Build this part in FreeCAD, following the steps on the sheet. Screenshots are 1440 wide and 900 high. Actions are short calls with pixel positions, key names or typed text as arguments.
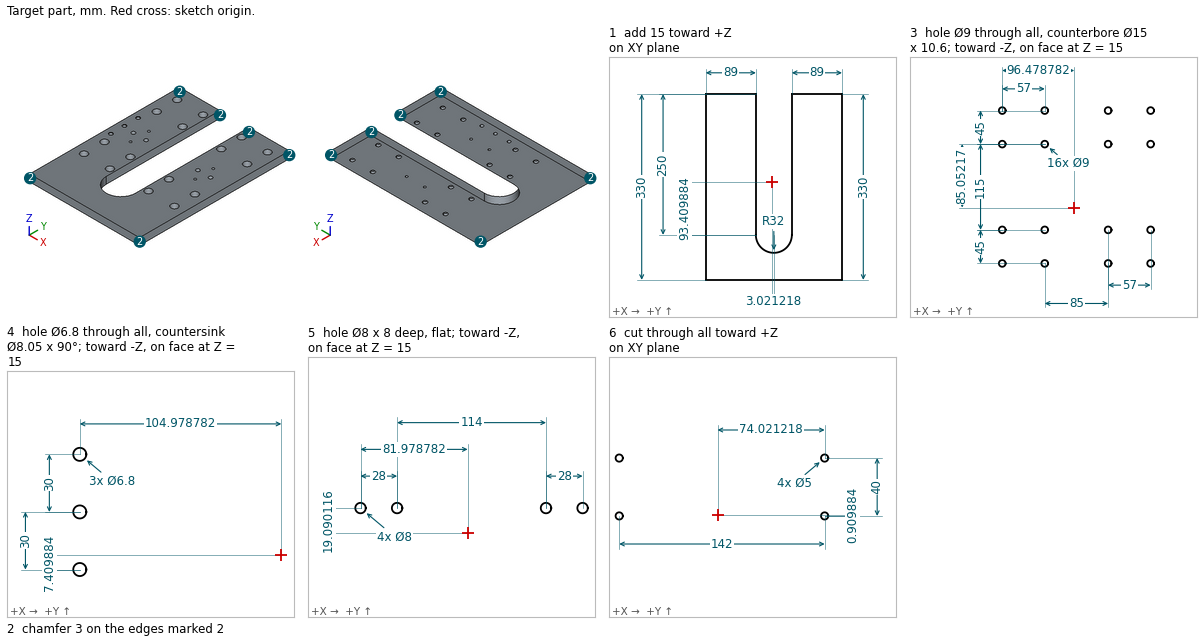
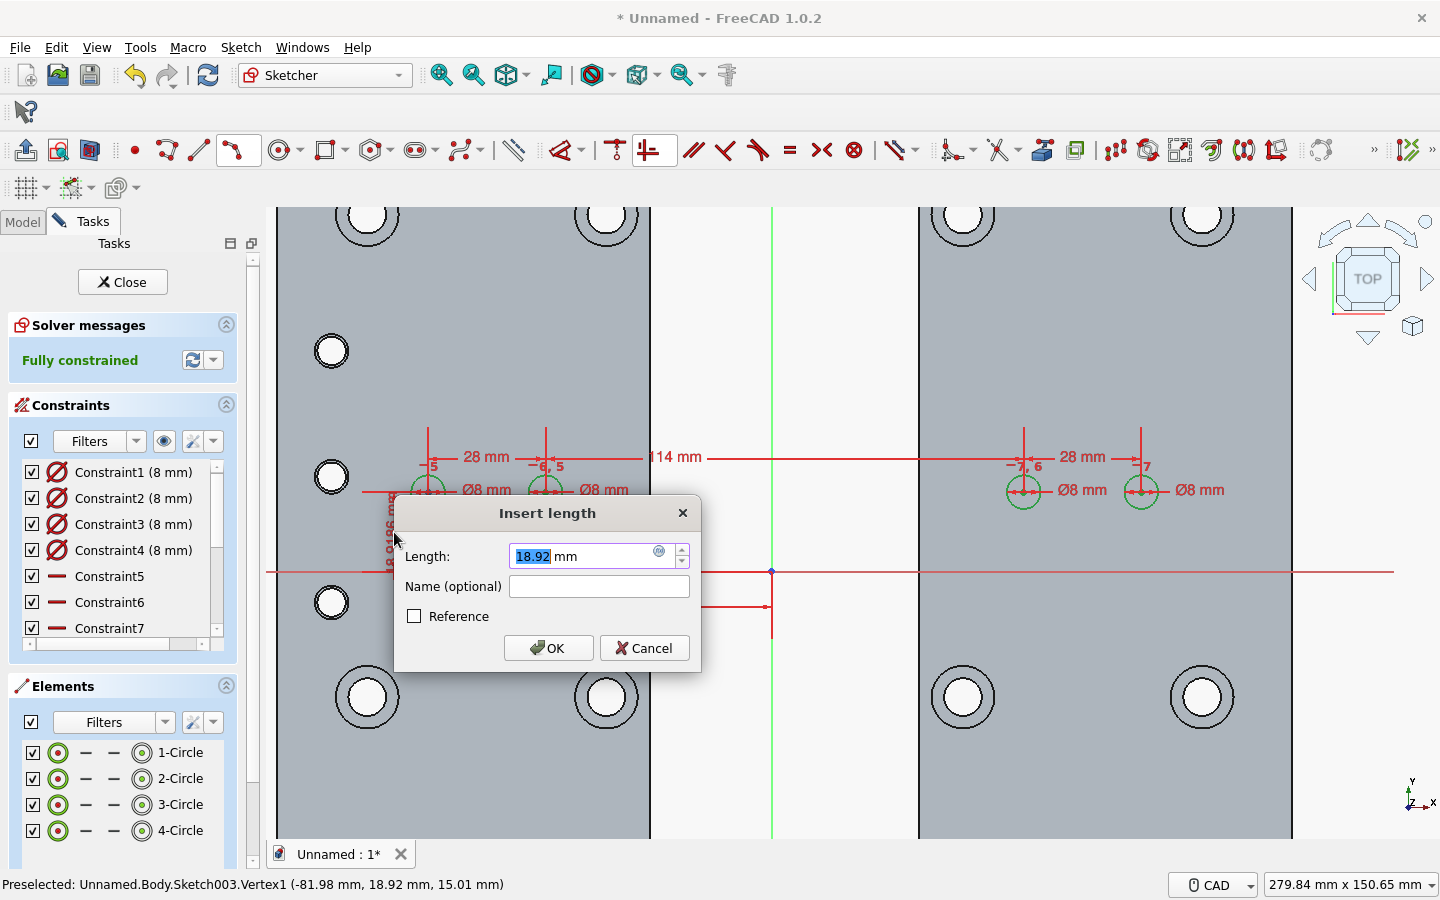
text(19.090116)
key(Return)
key(Escape)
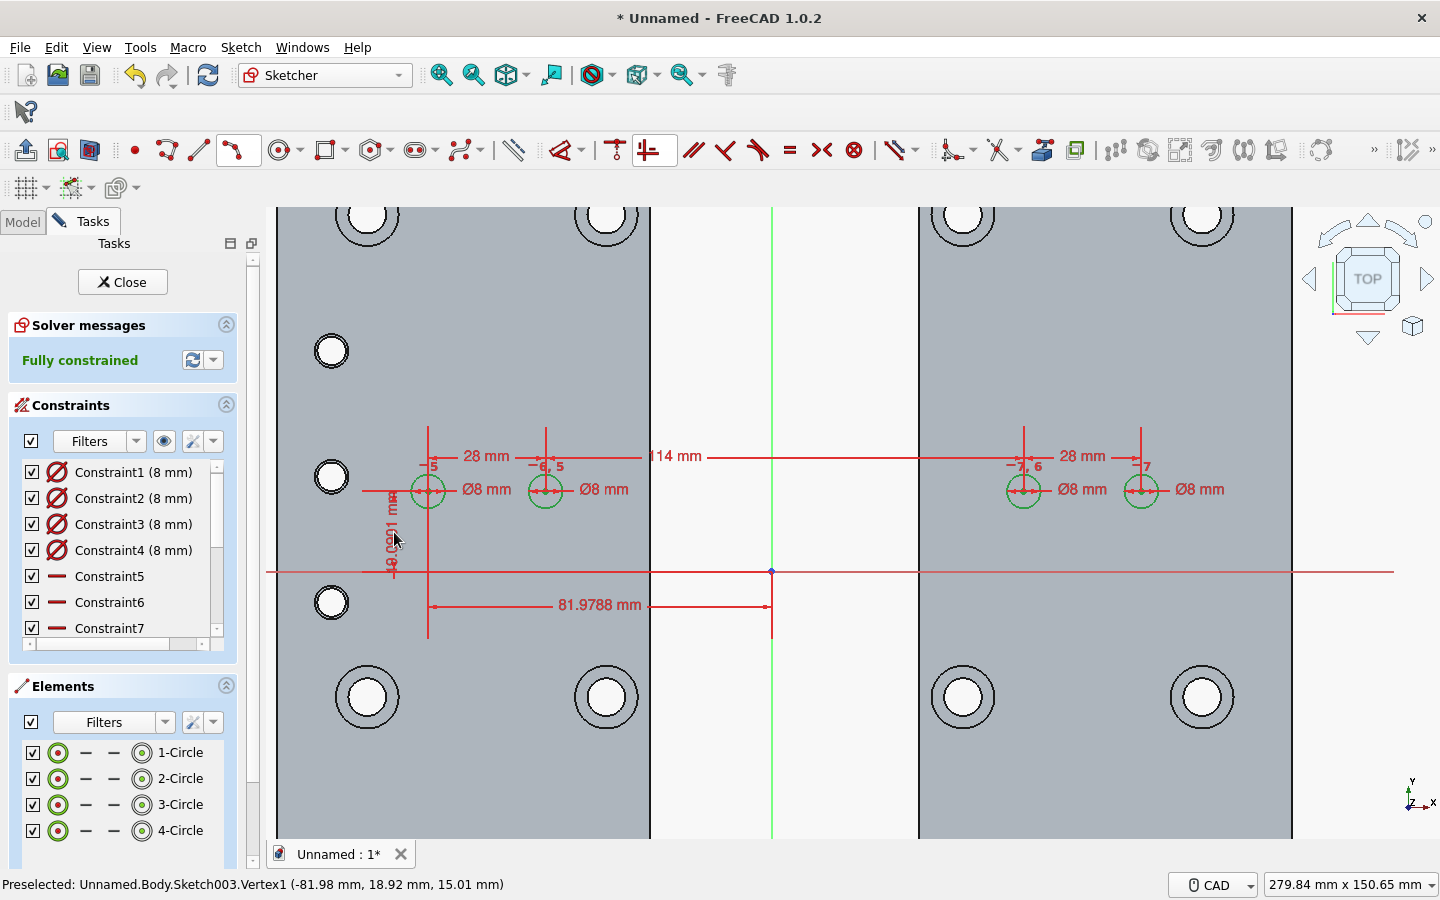
click(123, 282)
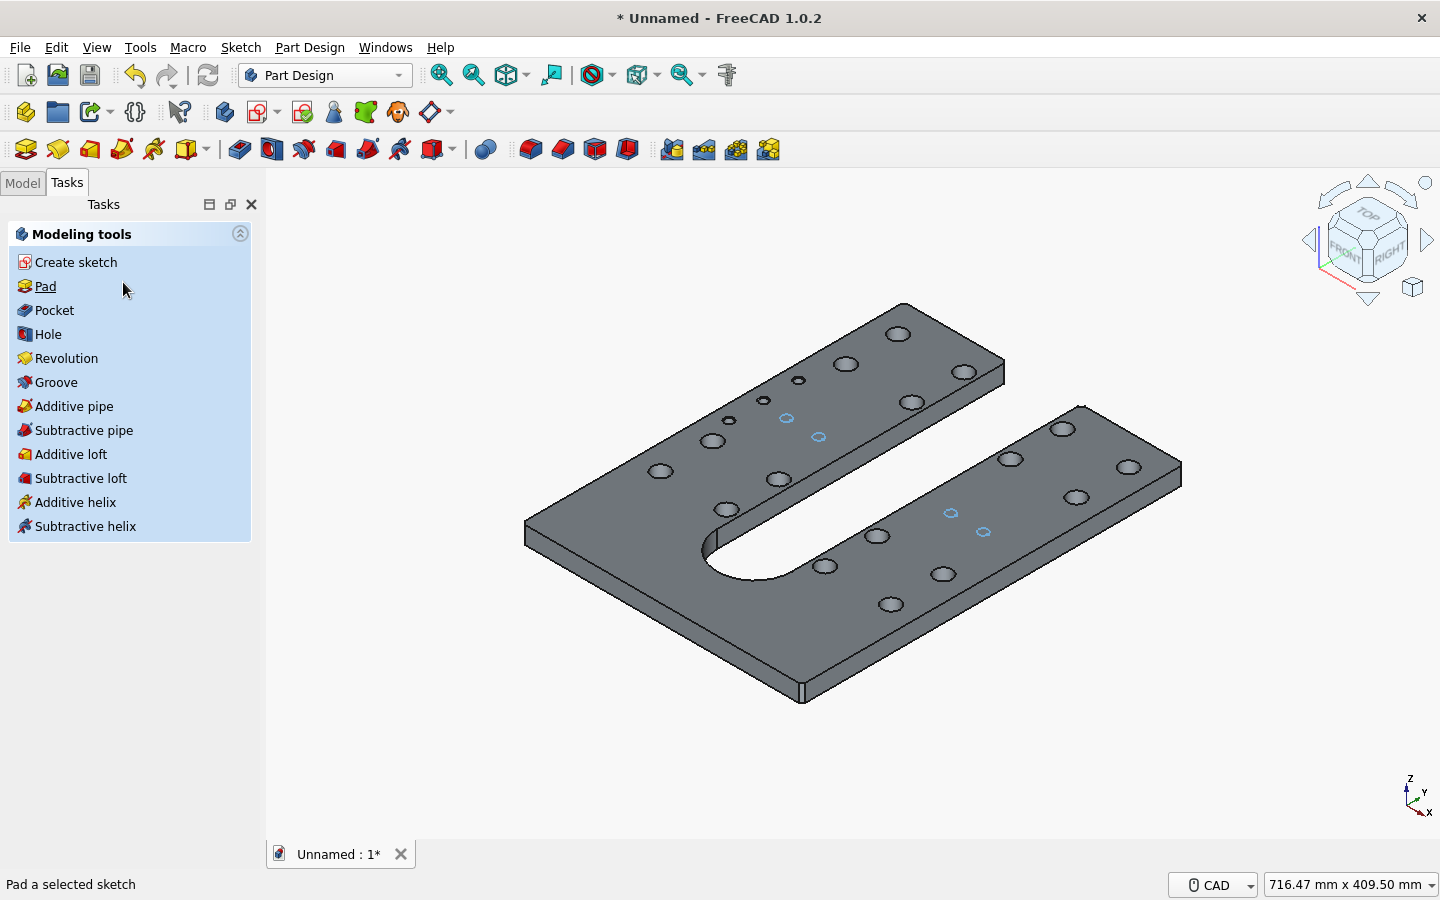
click(272, 150)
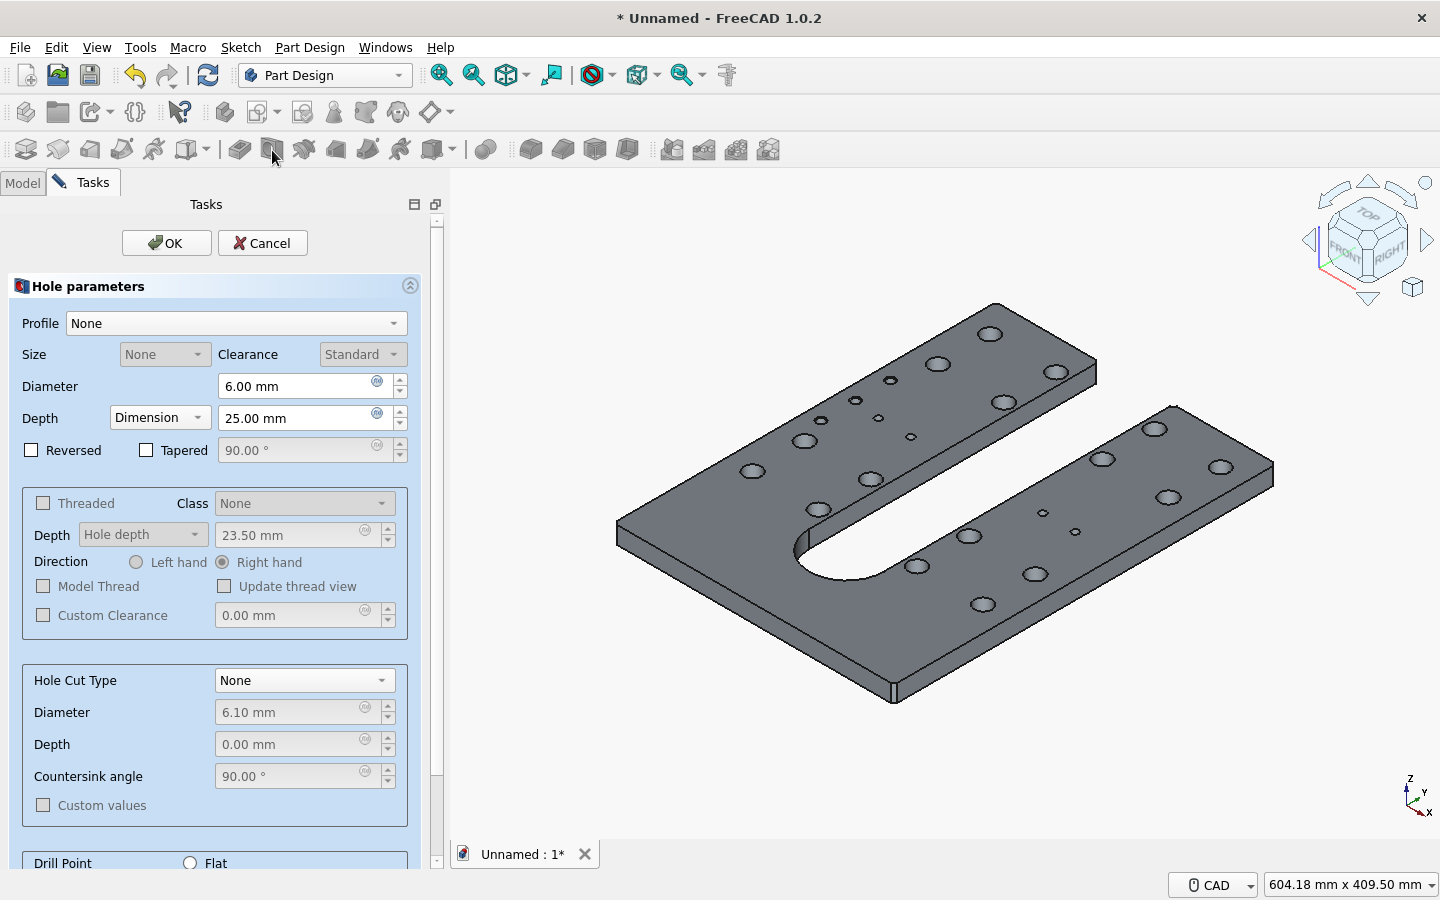
triple_click(305, 386)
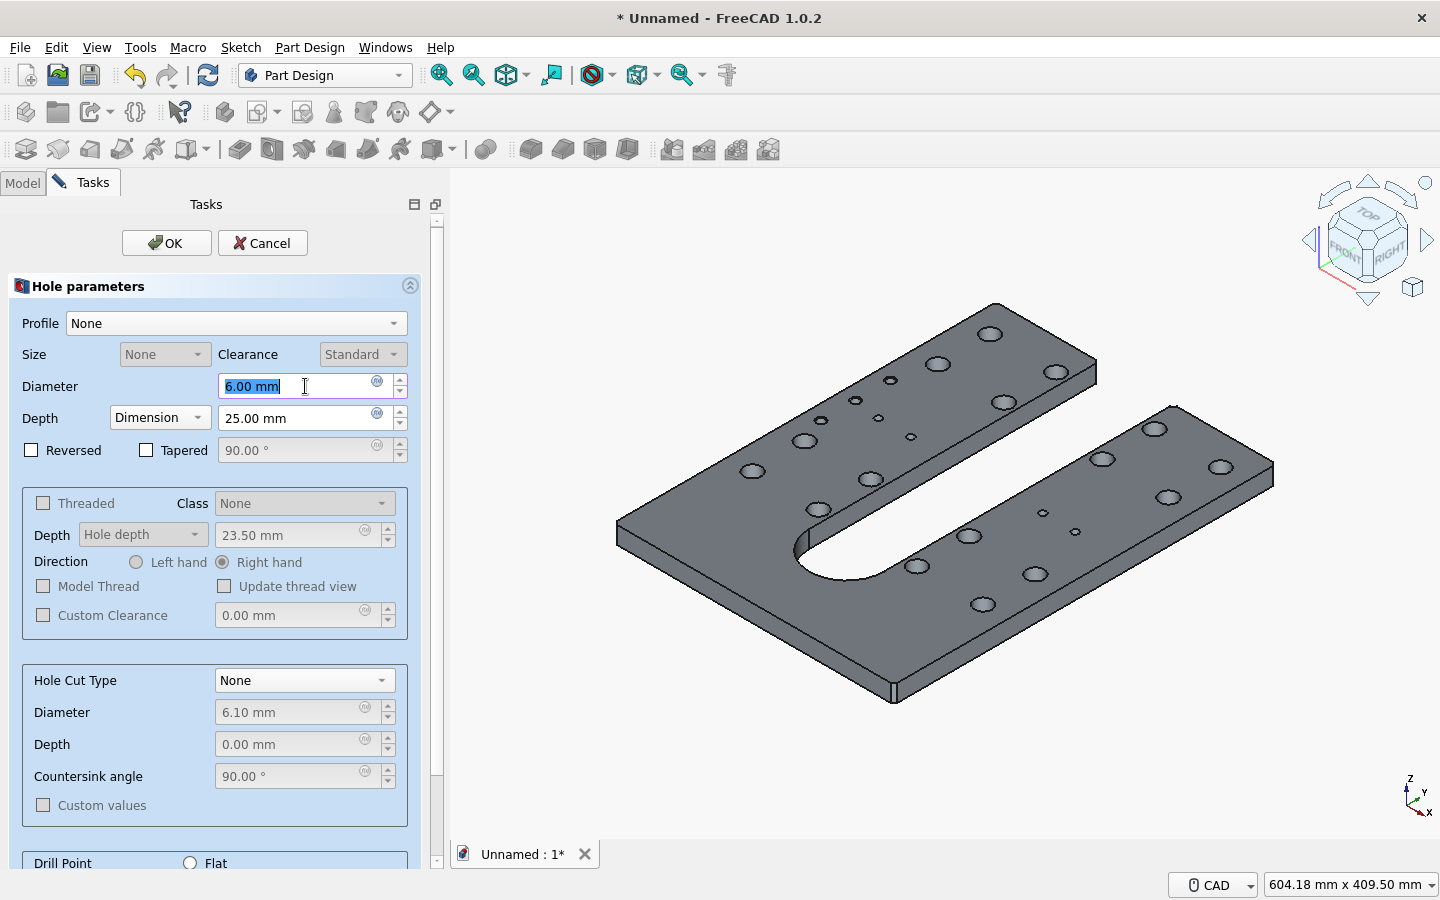
text(8)
key(Tab)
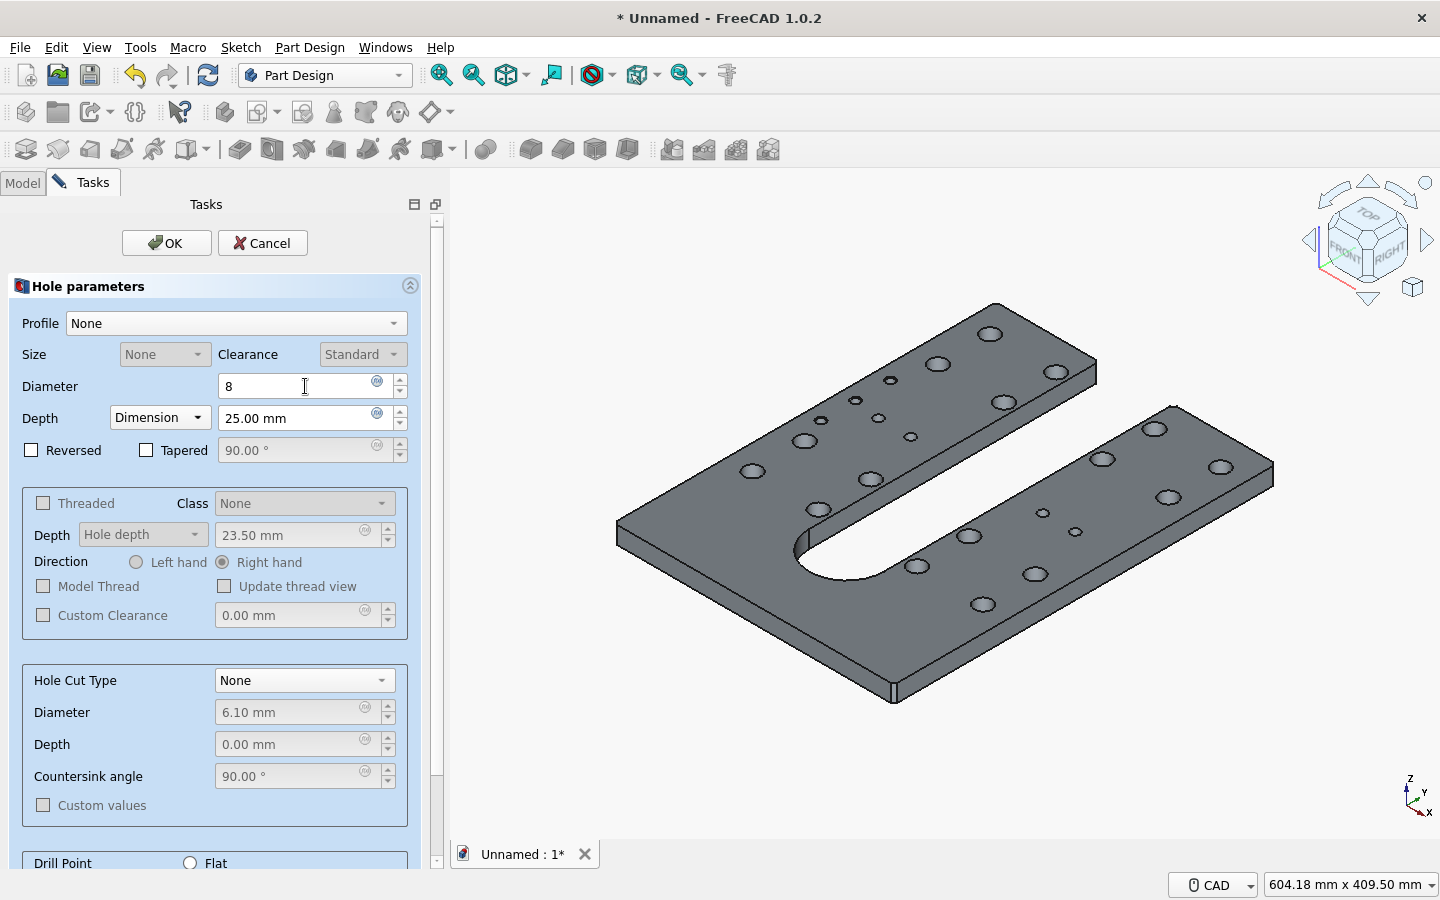
triple_click(305, 418)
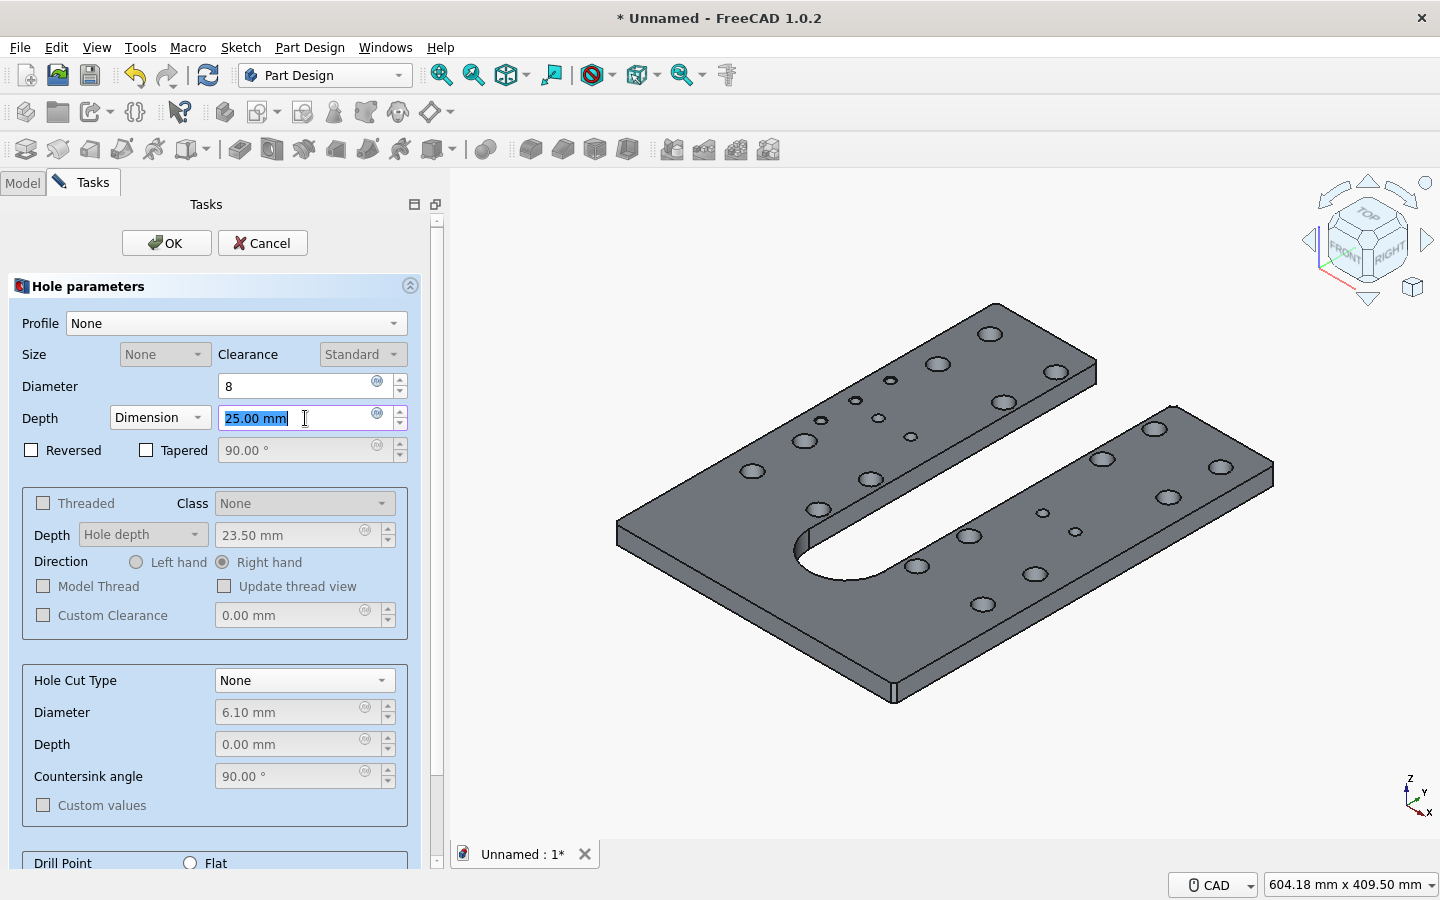
text(8)
key(Tab)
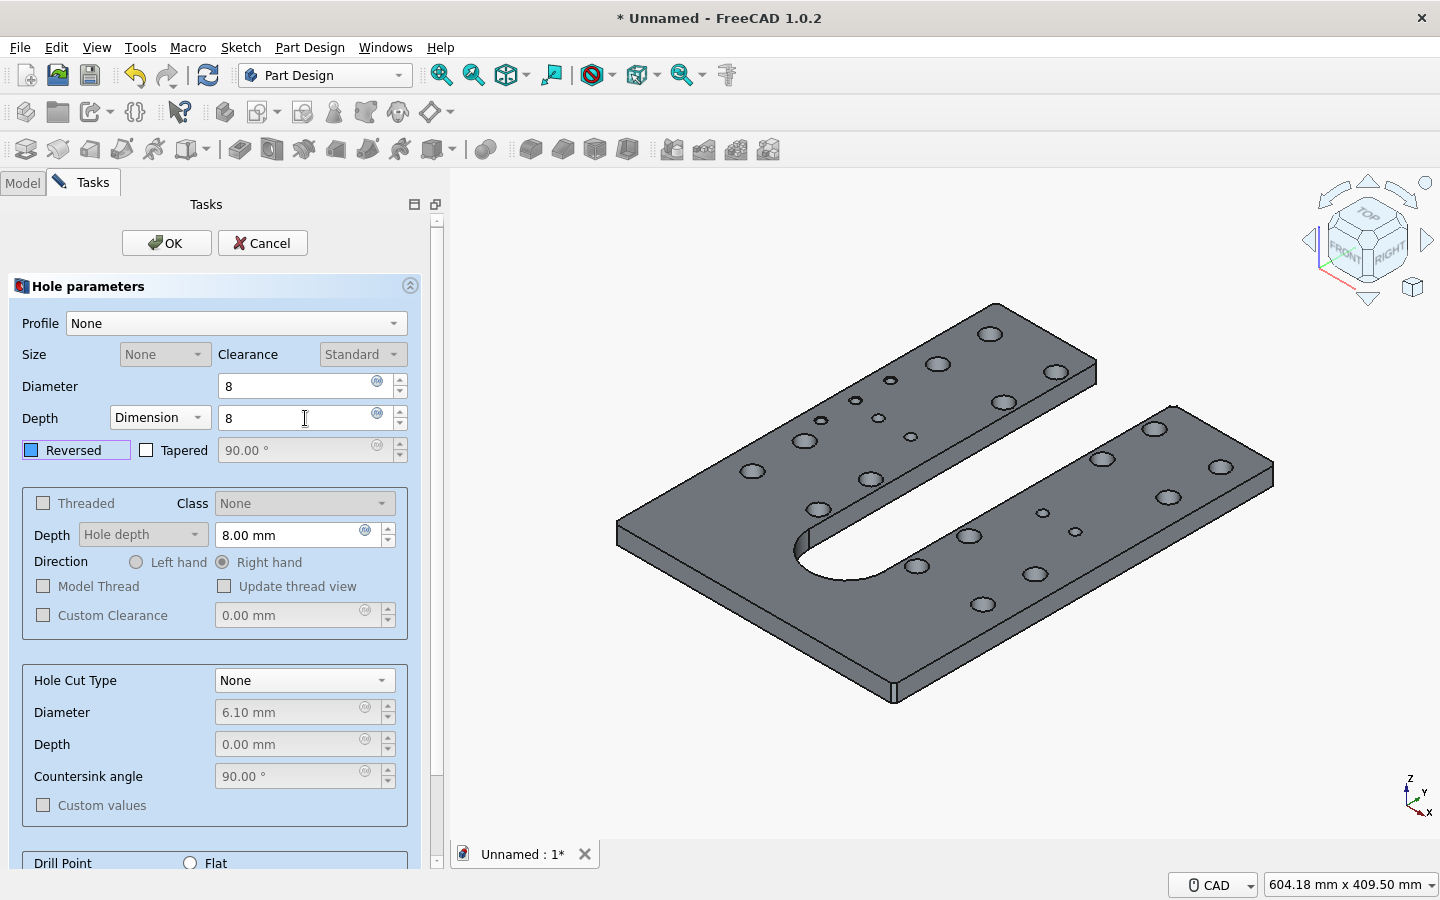
scroll(437, 541, down, 2)